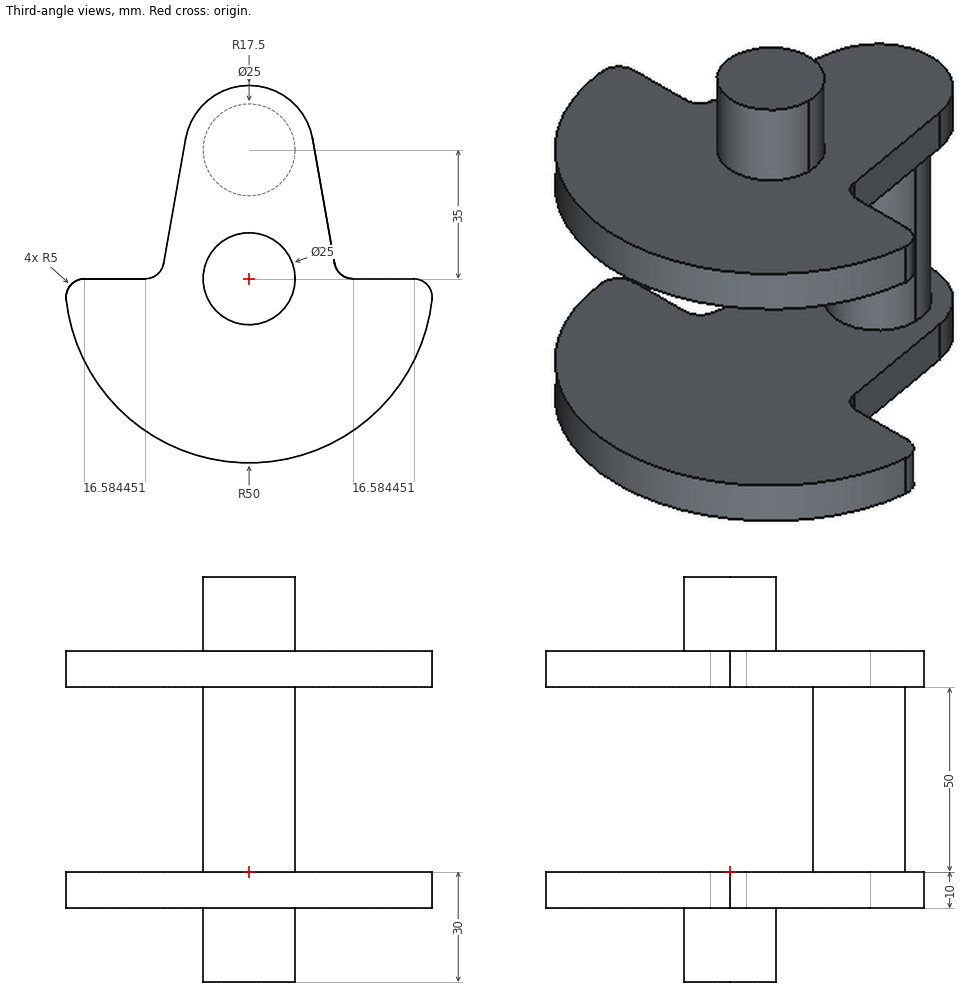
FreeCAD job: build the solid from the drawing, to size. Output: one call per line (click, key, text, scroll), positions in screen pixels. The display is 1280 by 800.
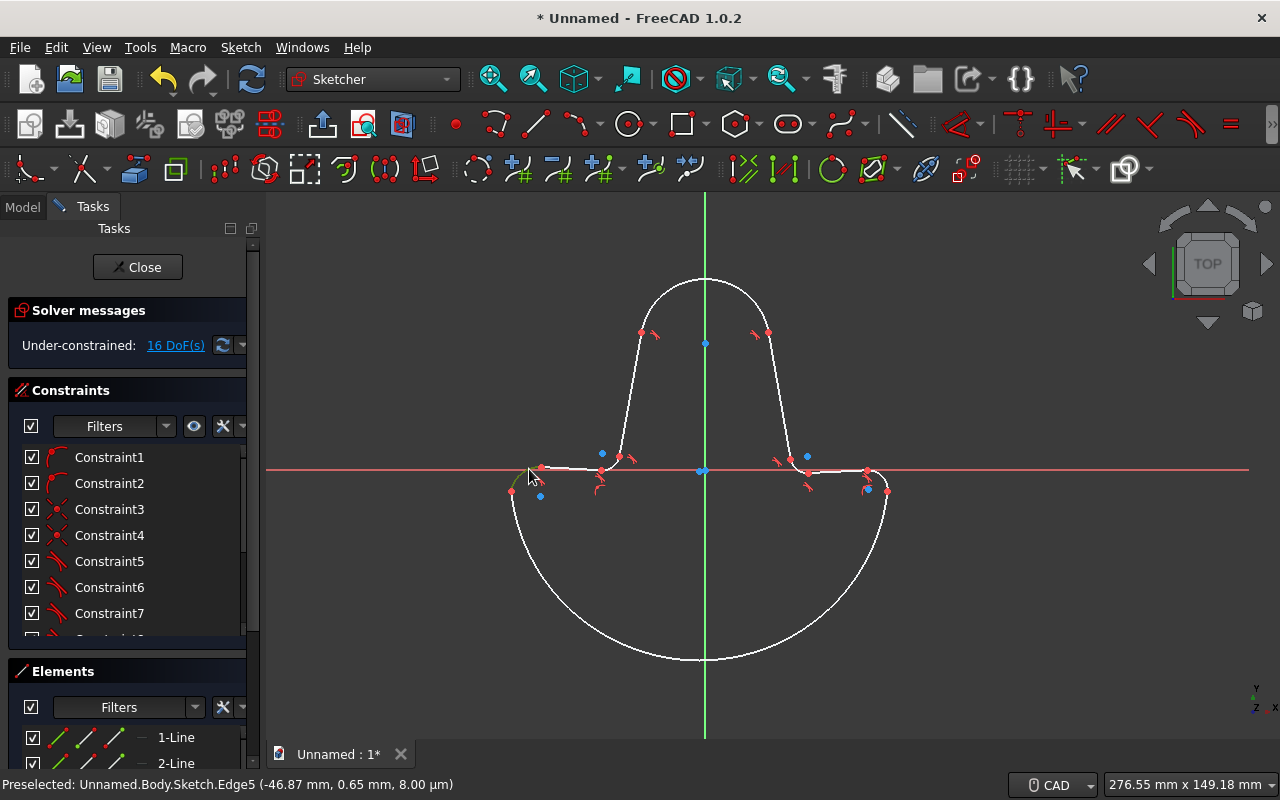
click(595, 629)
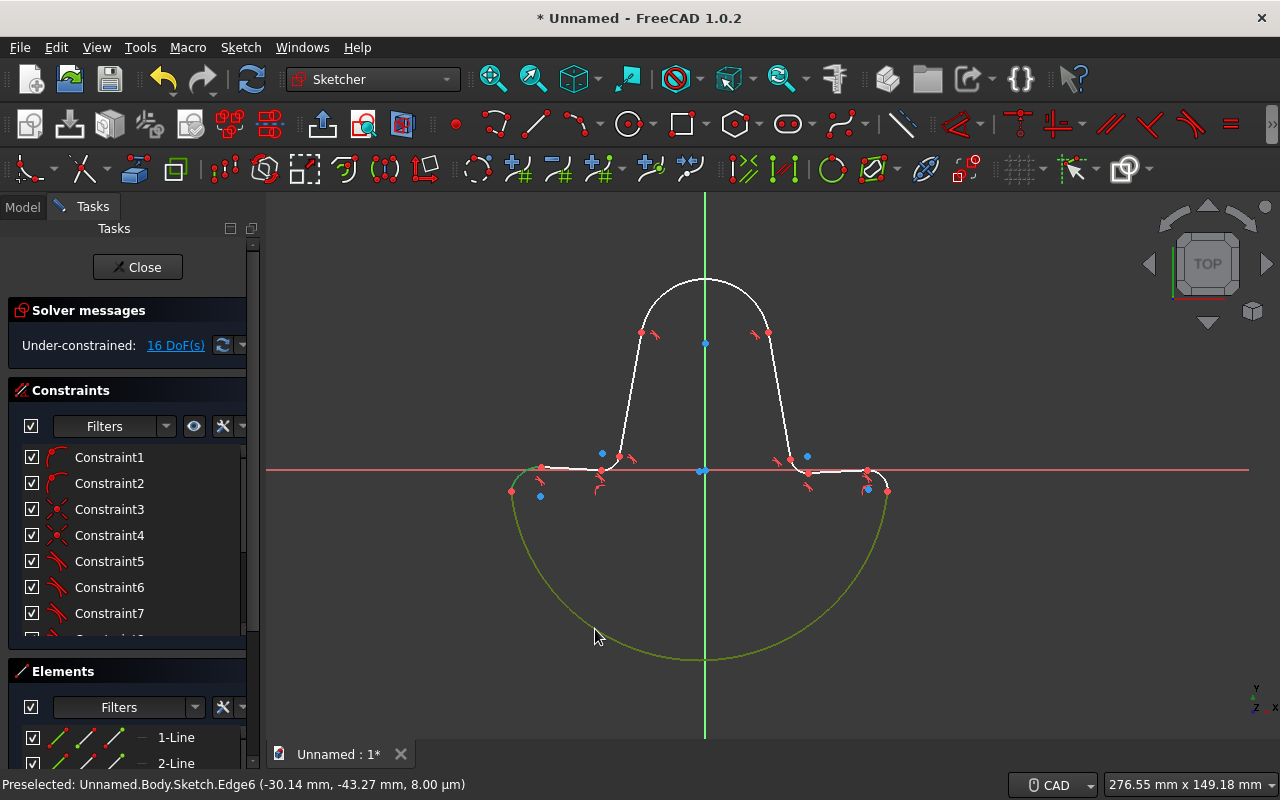
key(t)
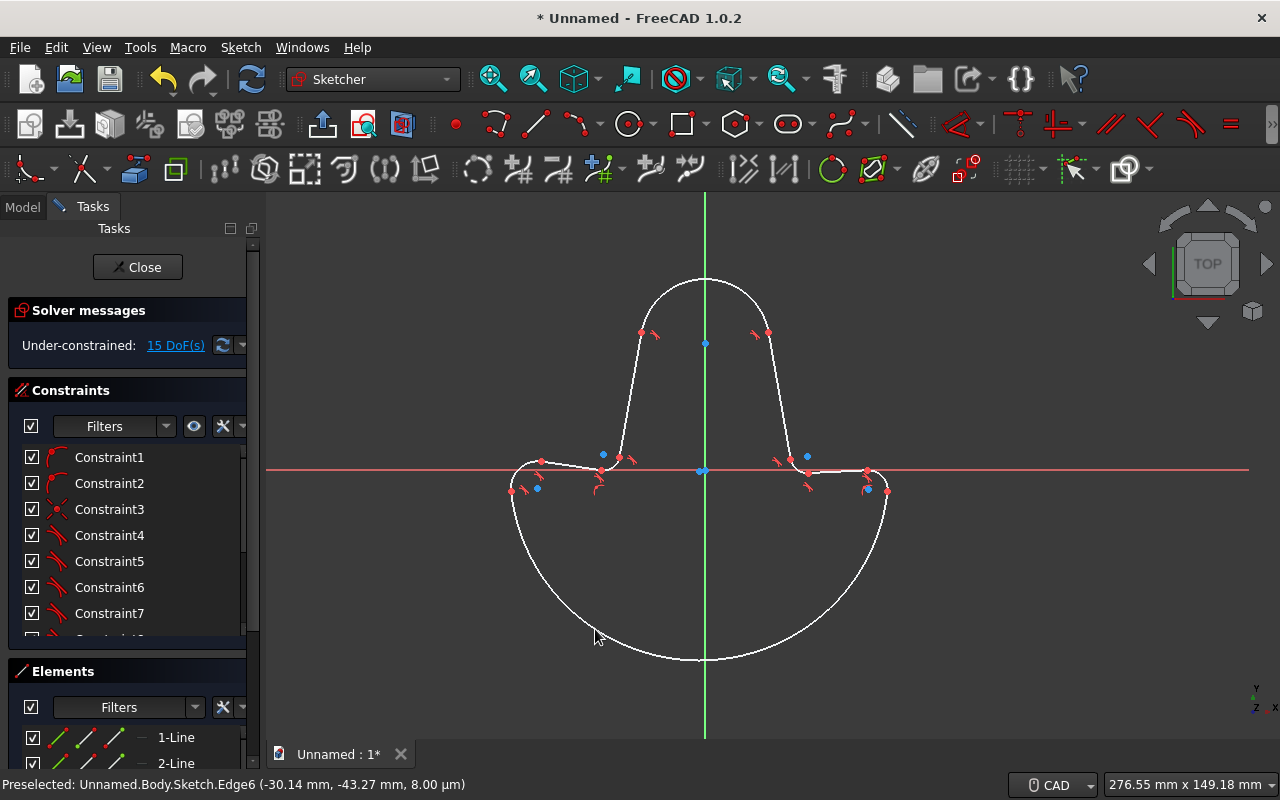
click(595, 629)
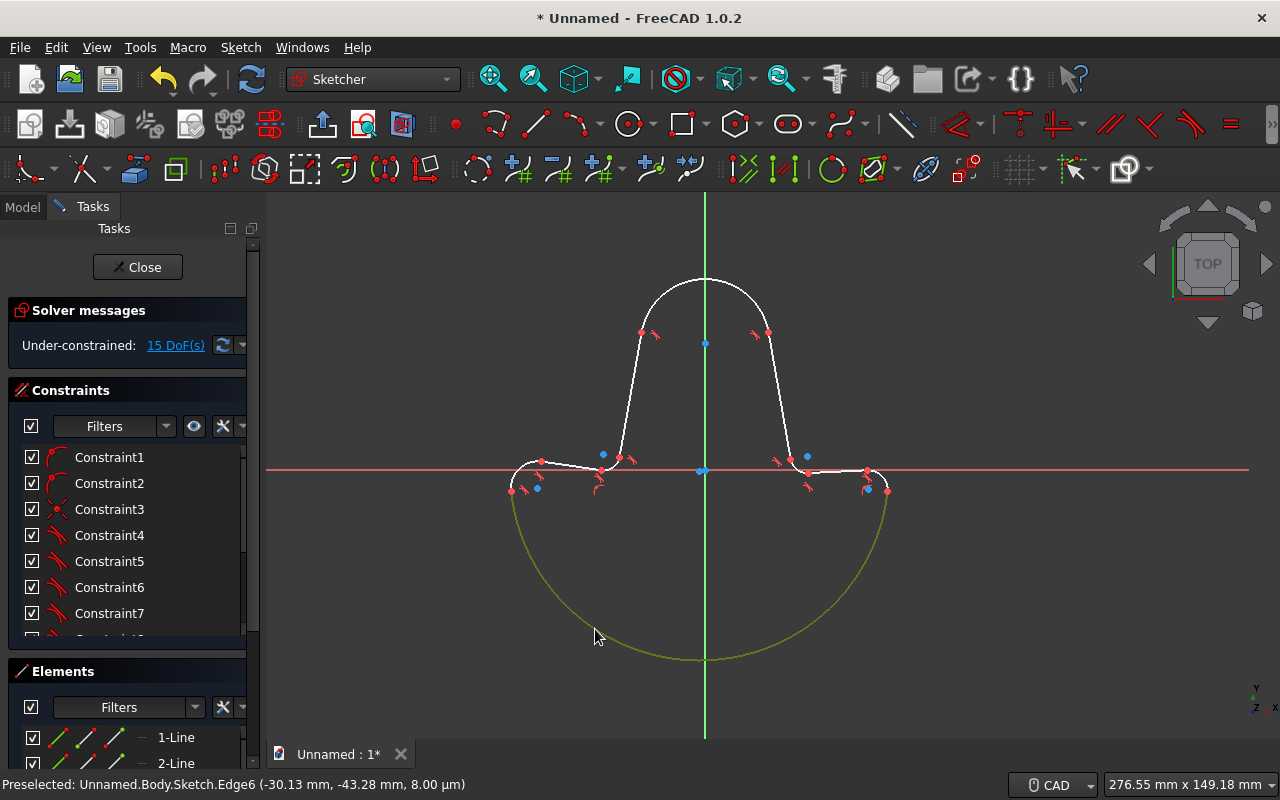
scroll(886, 481, up, 2)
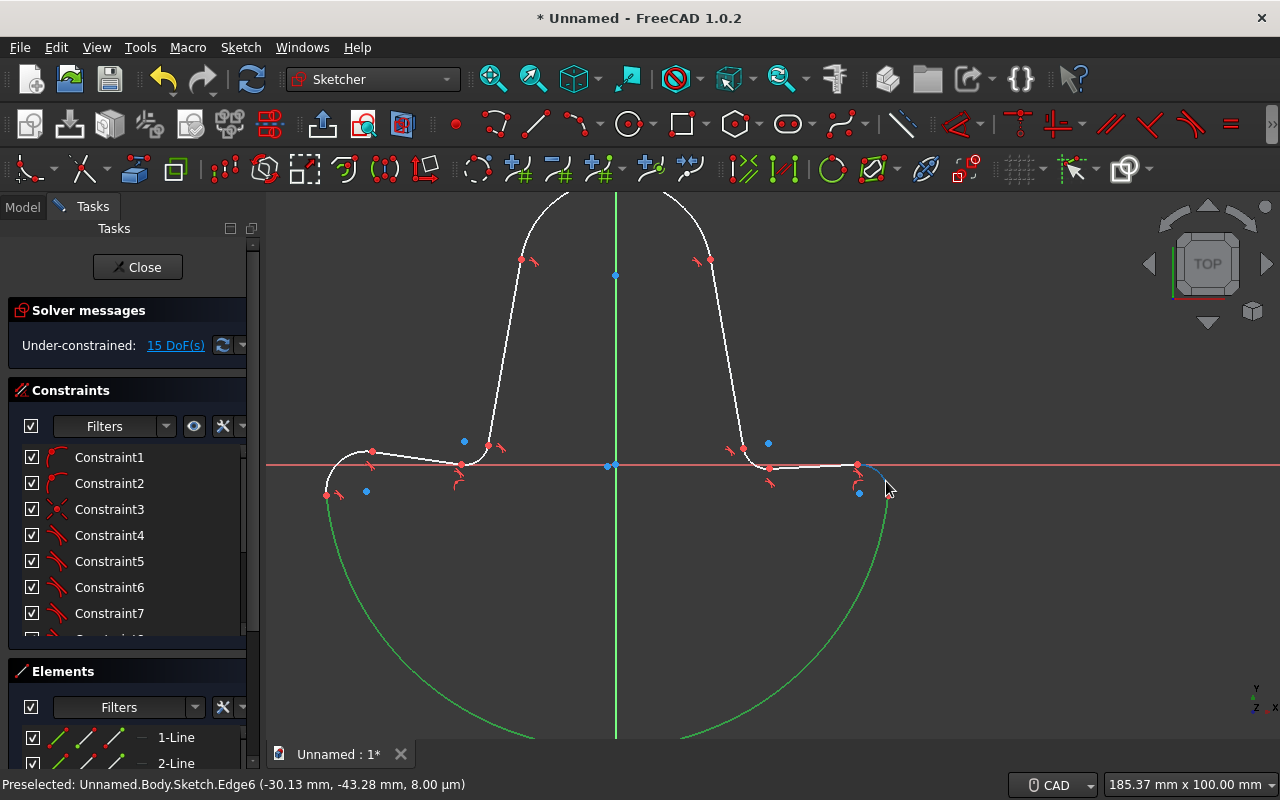
click(885, 481)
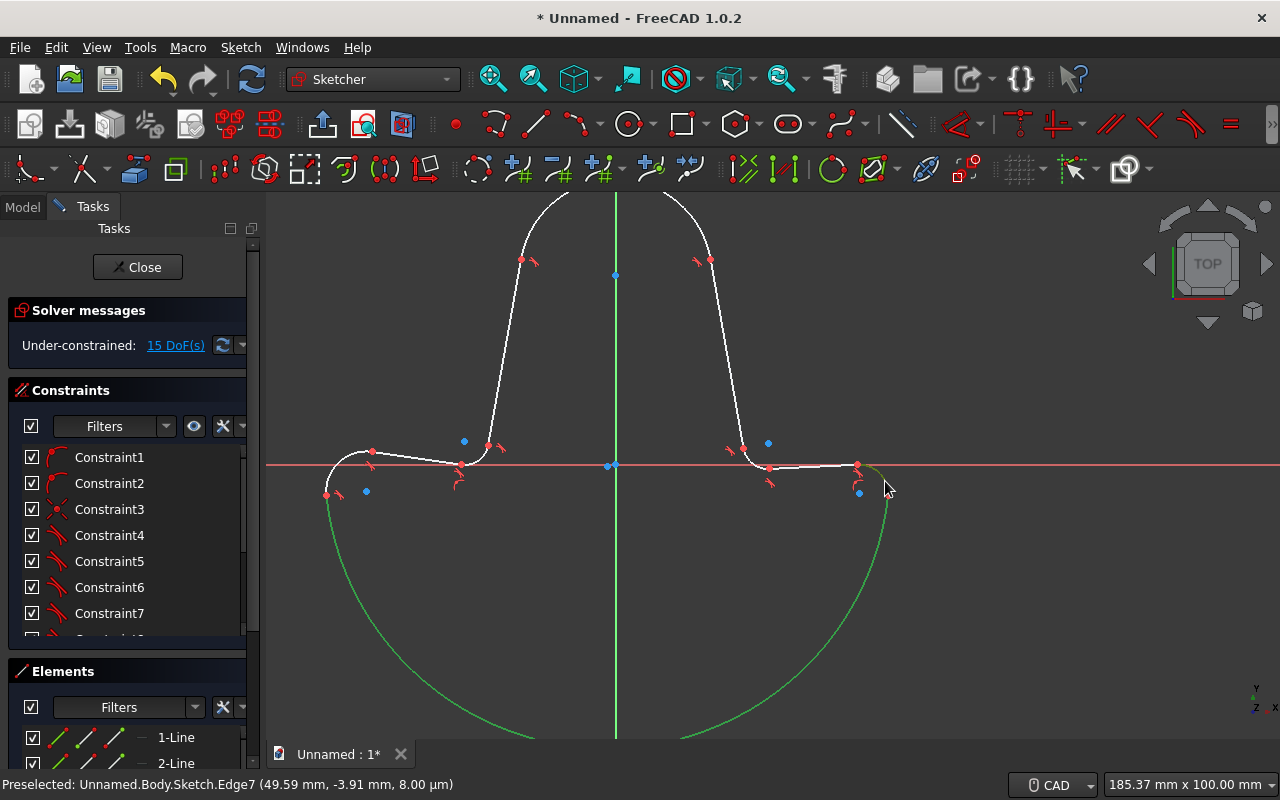
click(1192, 124)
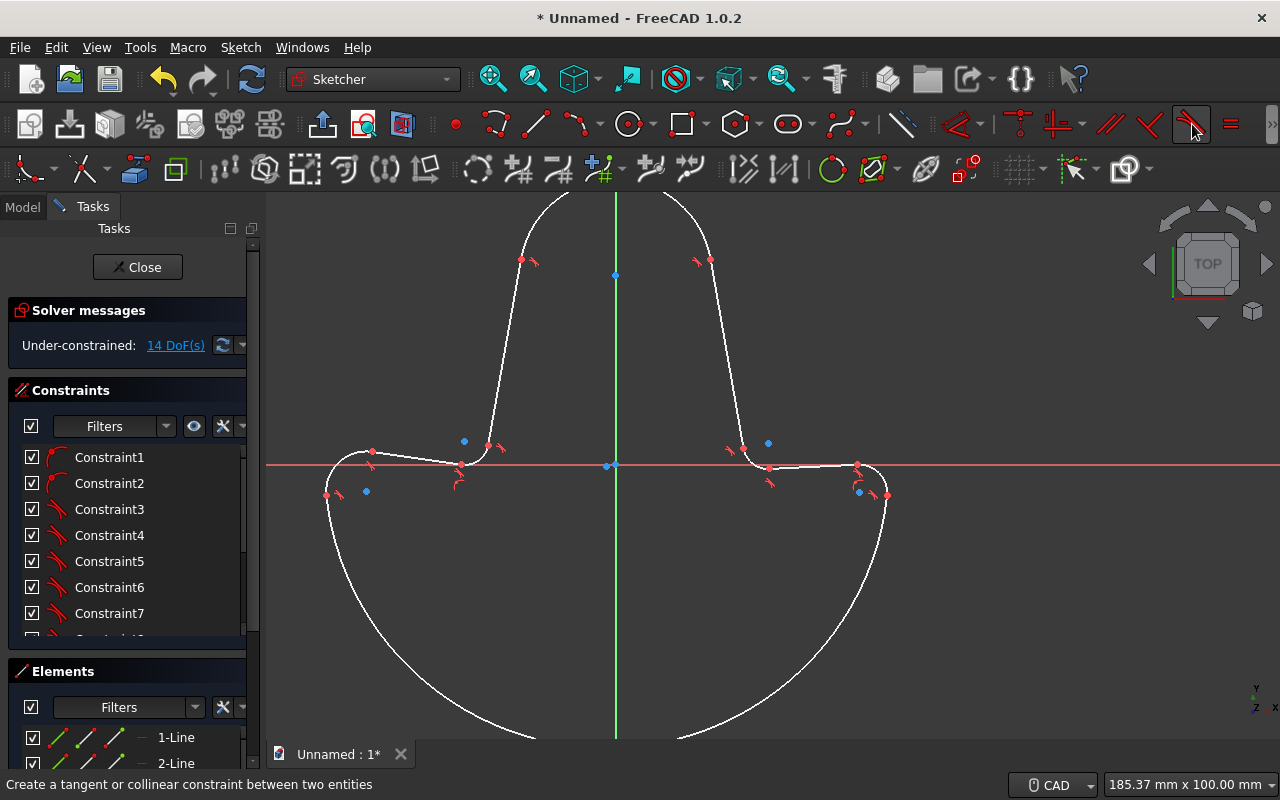
click(435, 461)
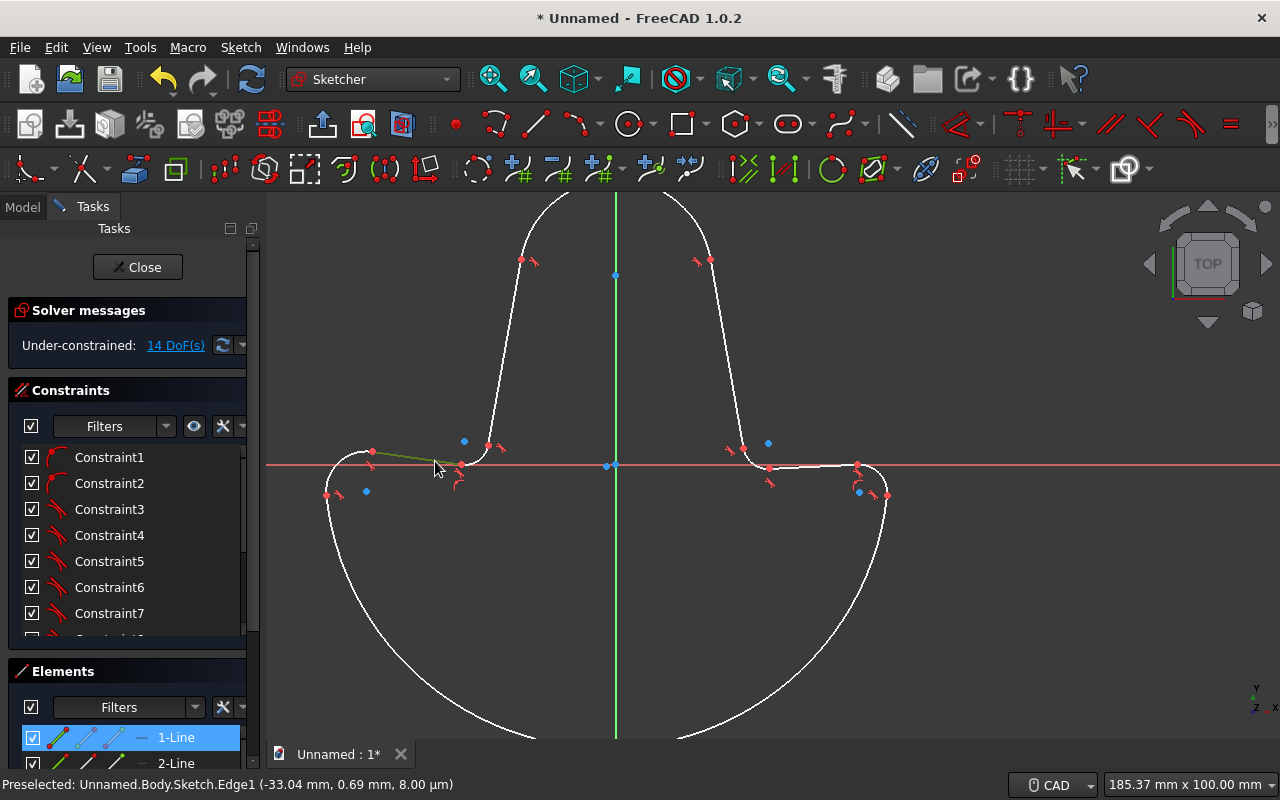
key(h)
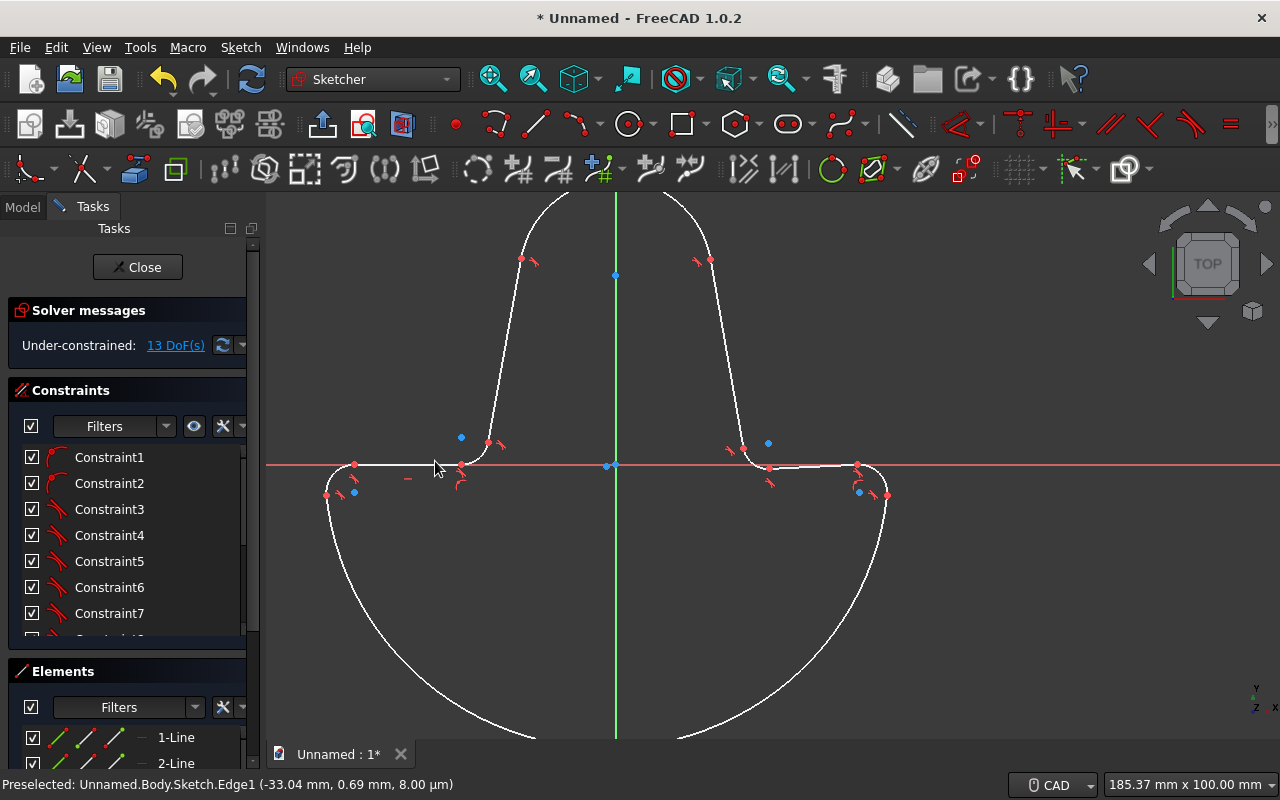
click(831, 466)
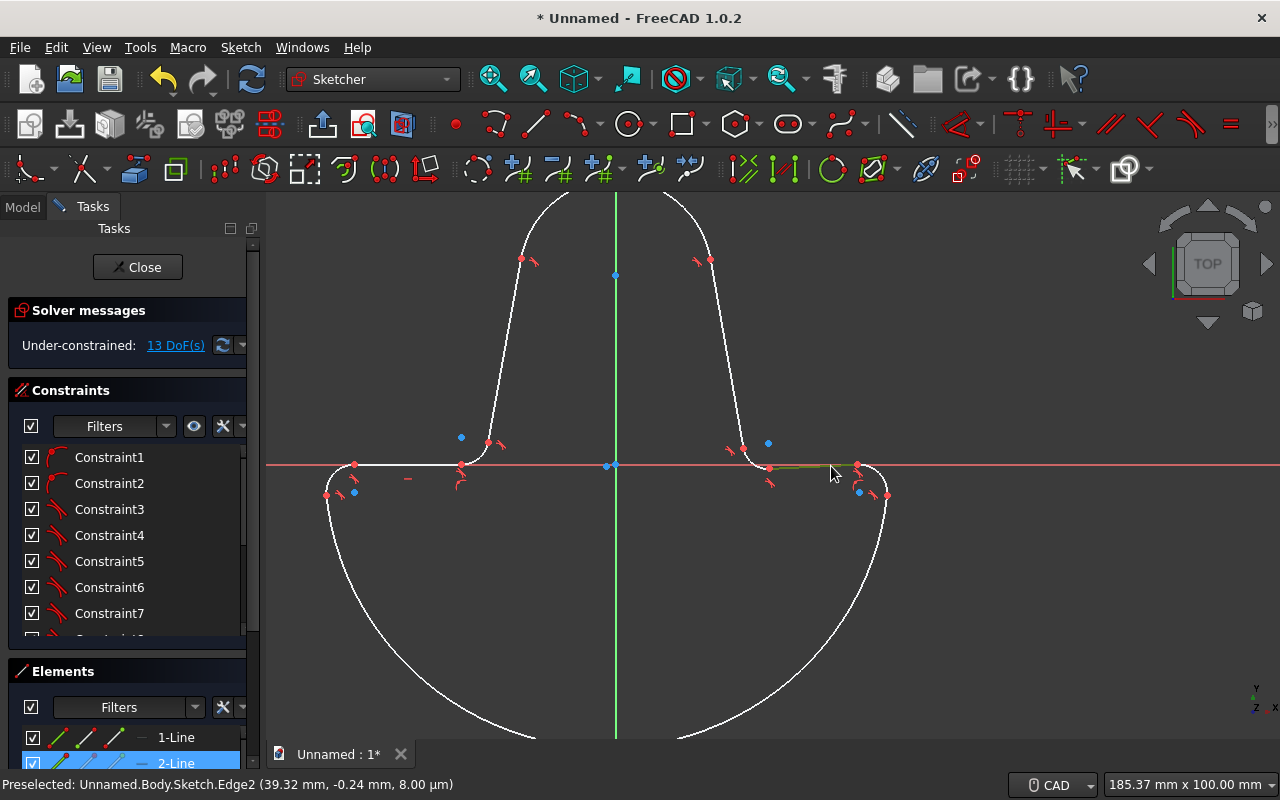
key(h)